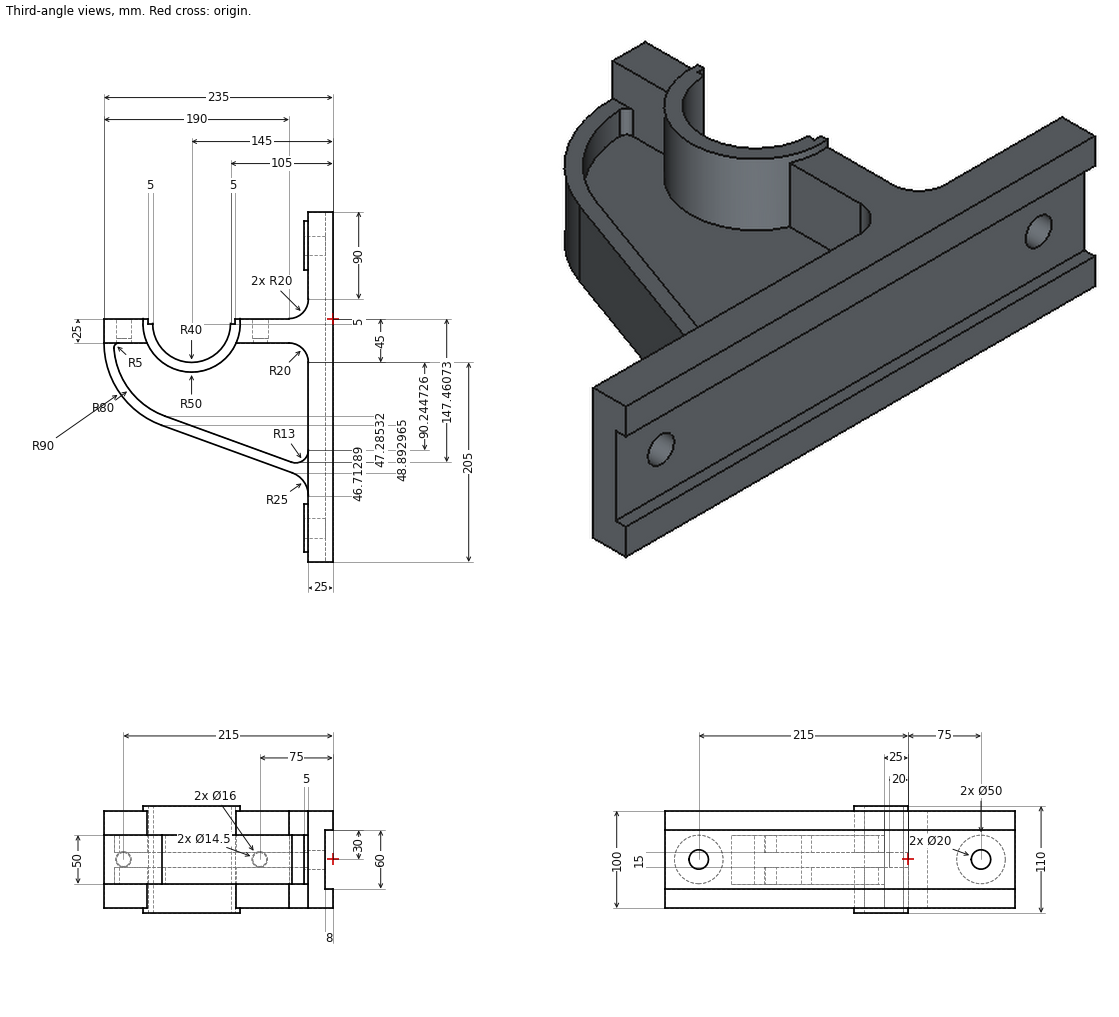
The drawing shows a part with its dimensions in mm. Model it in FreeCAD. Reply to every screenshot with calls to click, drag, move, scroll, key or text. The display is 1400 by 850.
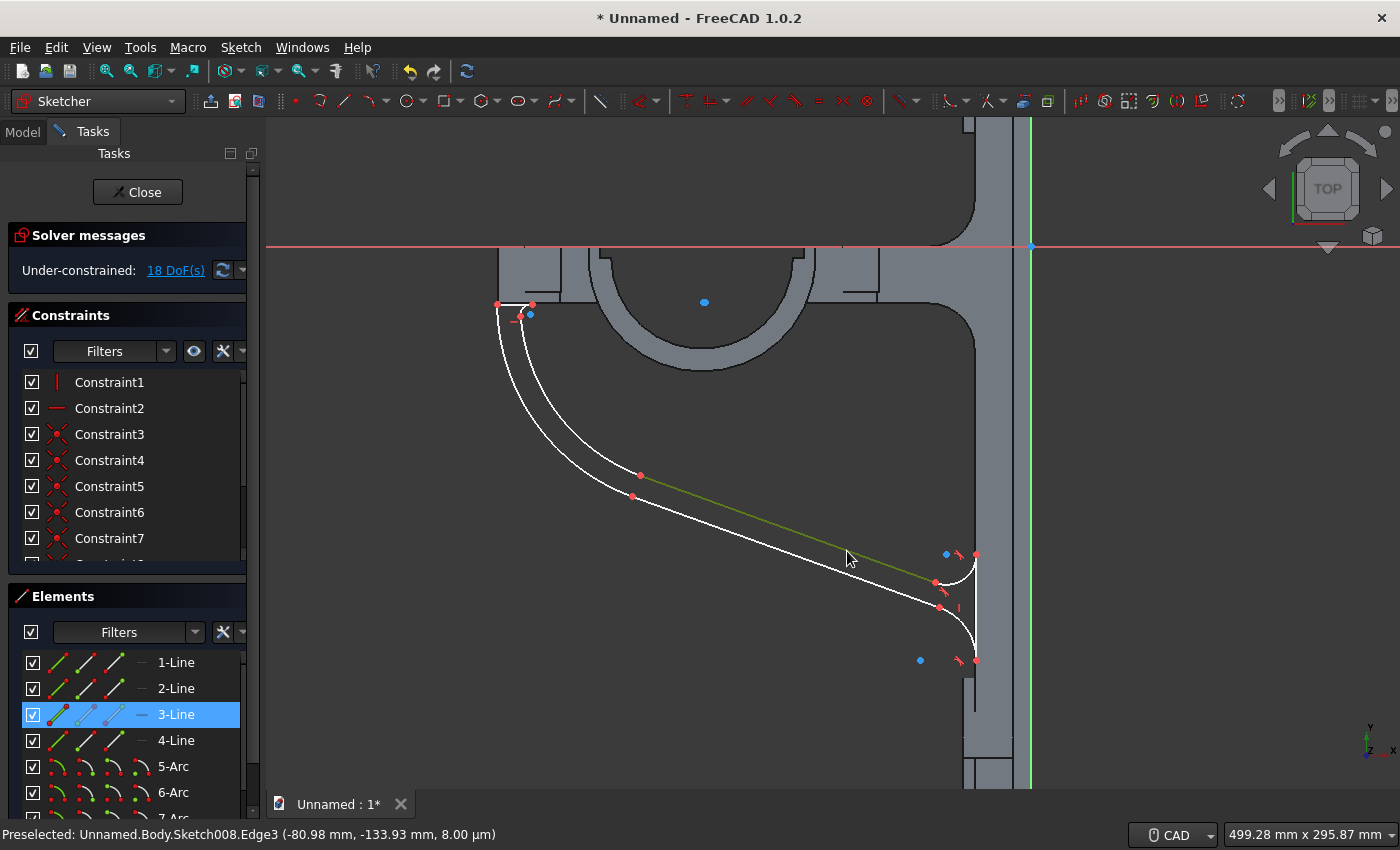
click(952, 584)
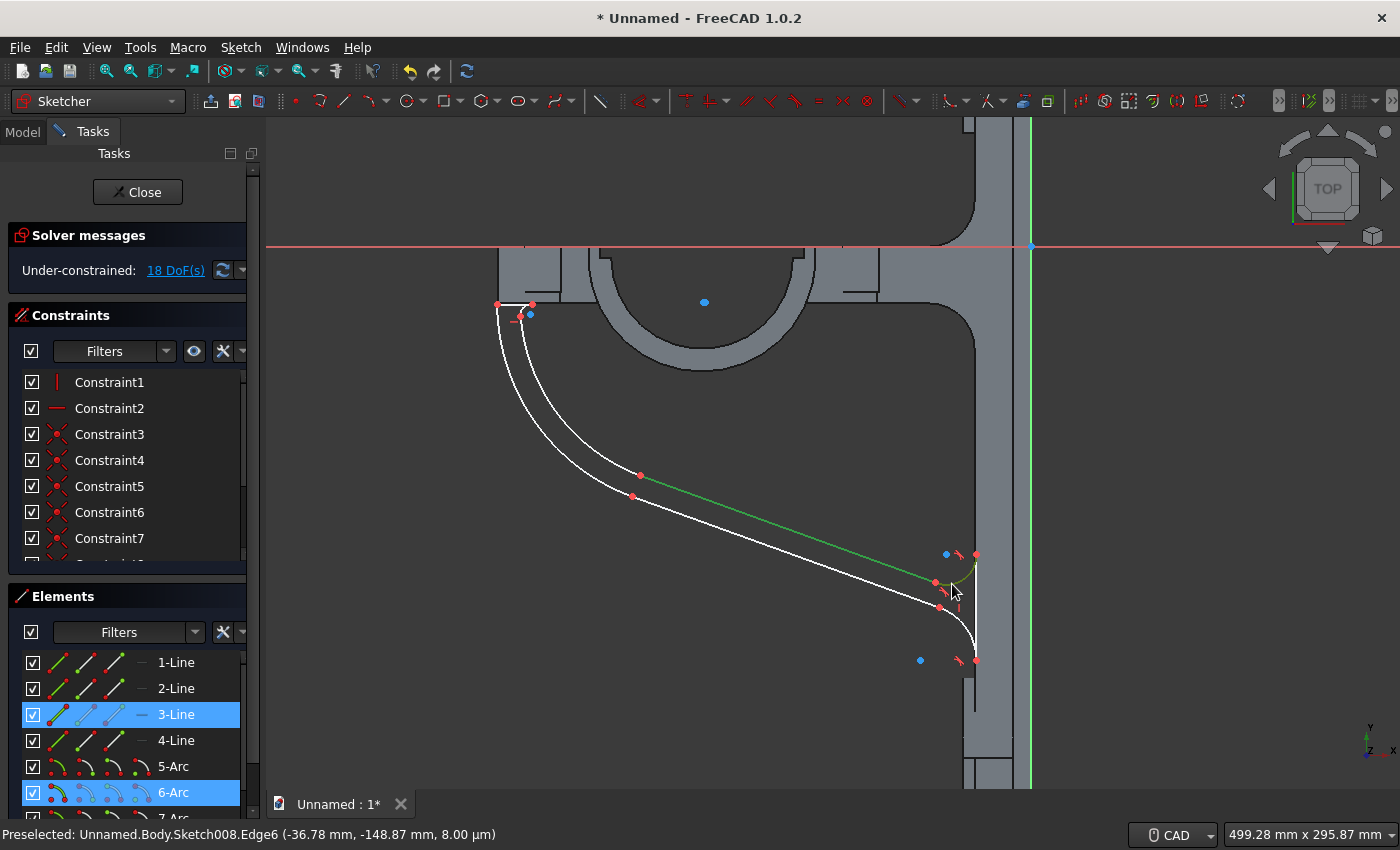
click(796, 102)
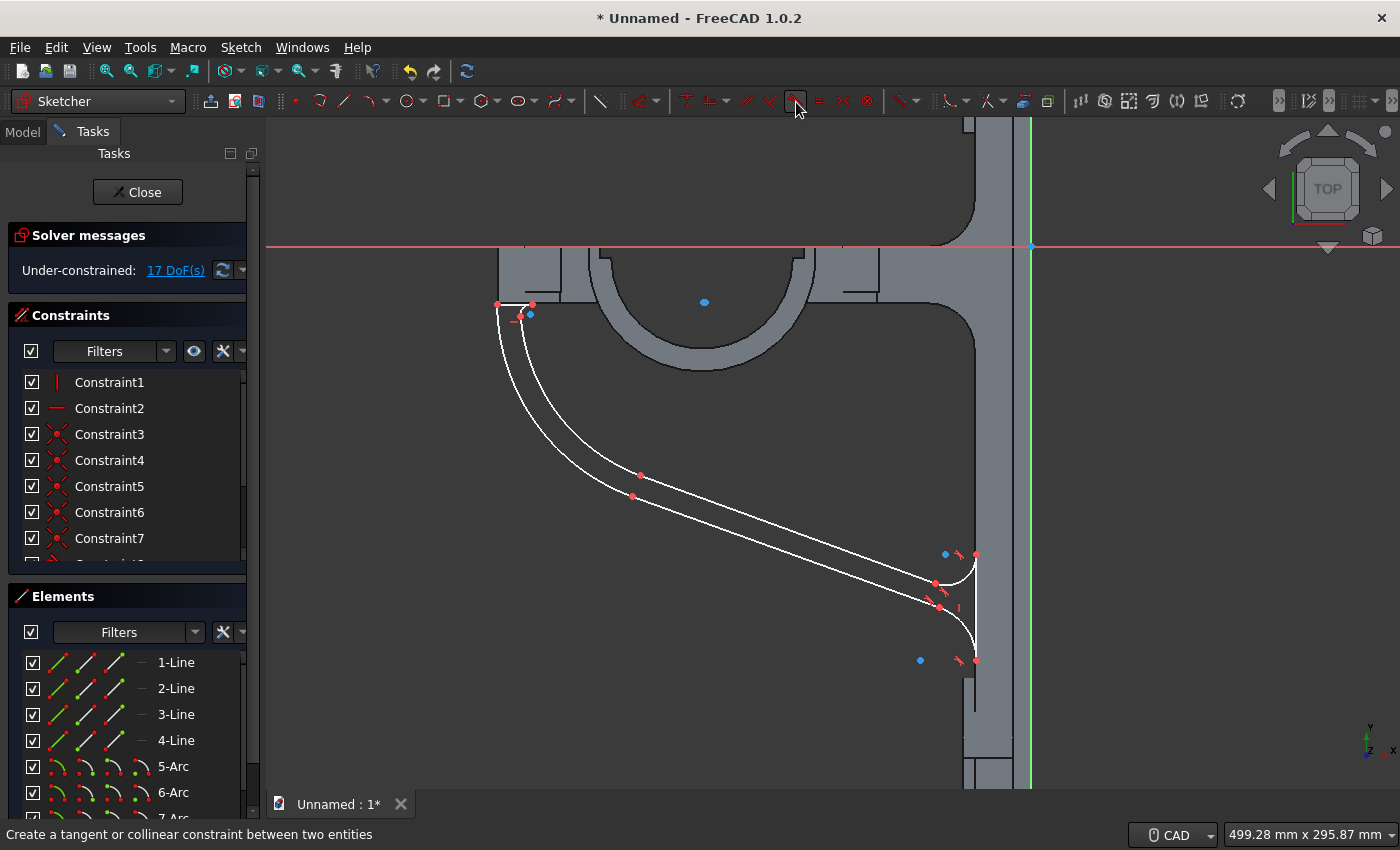
scroll(508, 305, up, 2)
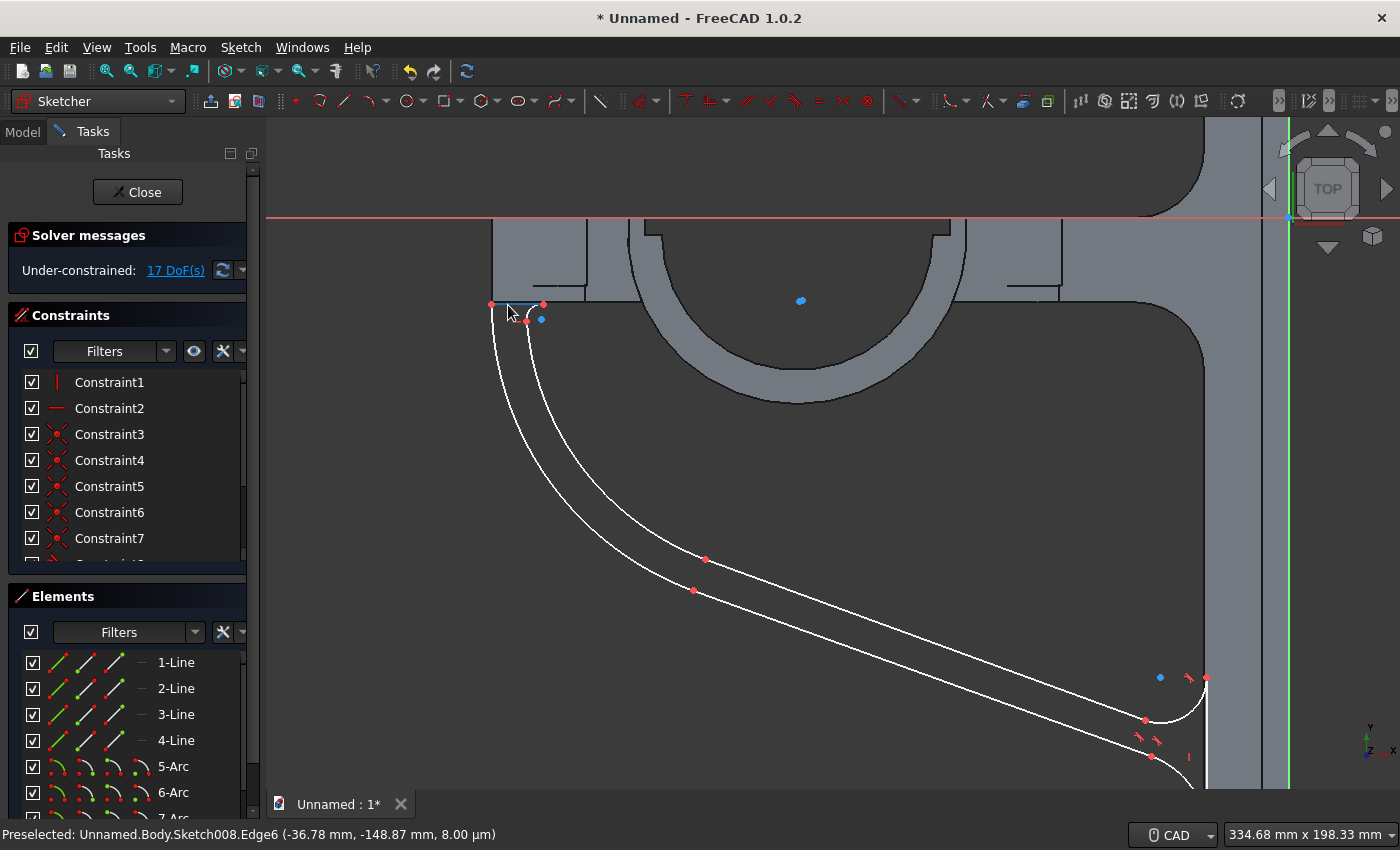
click(507, 304)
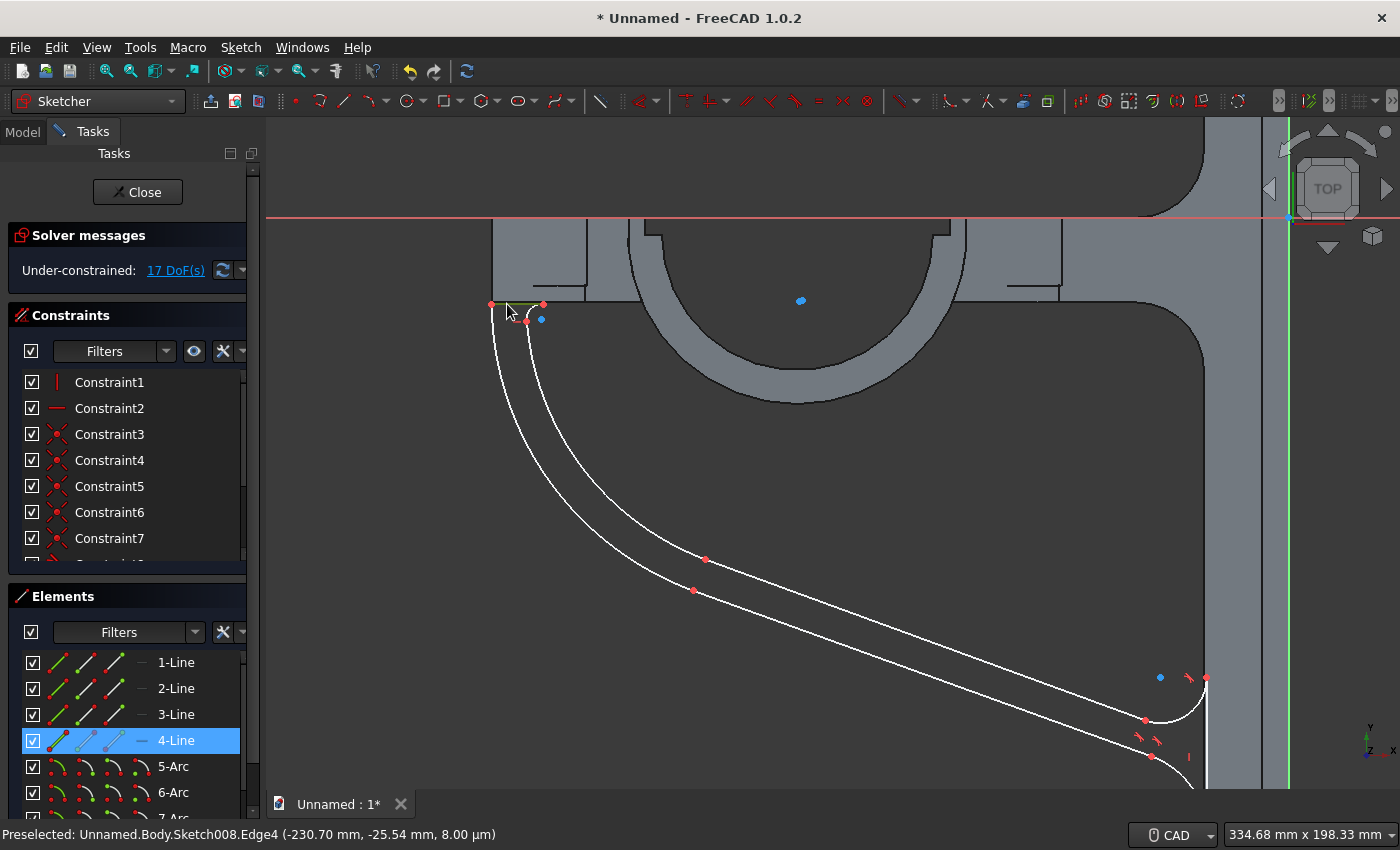
scroll(528, 314, up, 3)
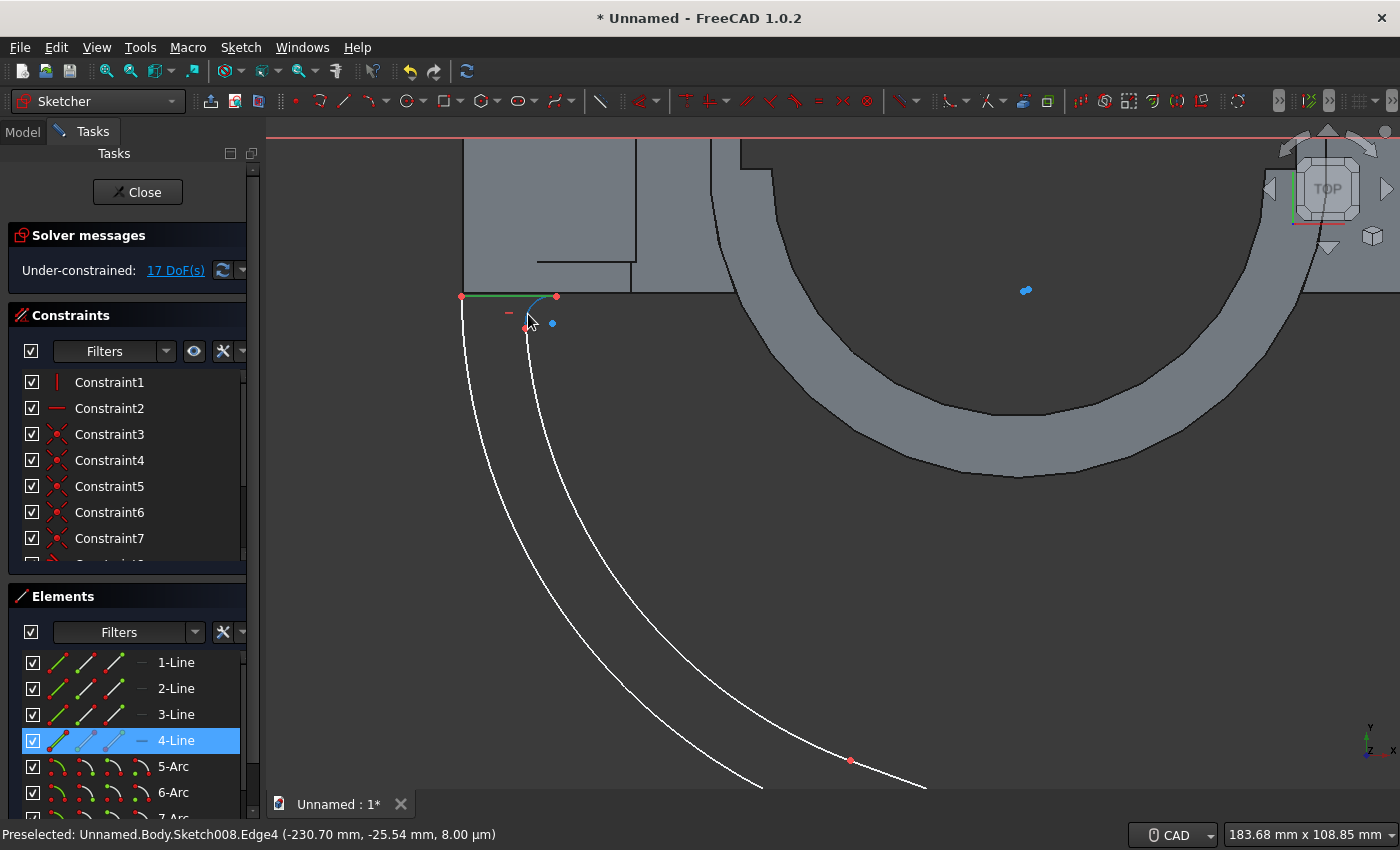
click(527, 313)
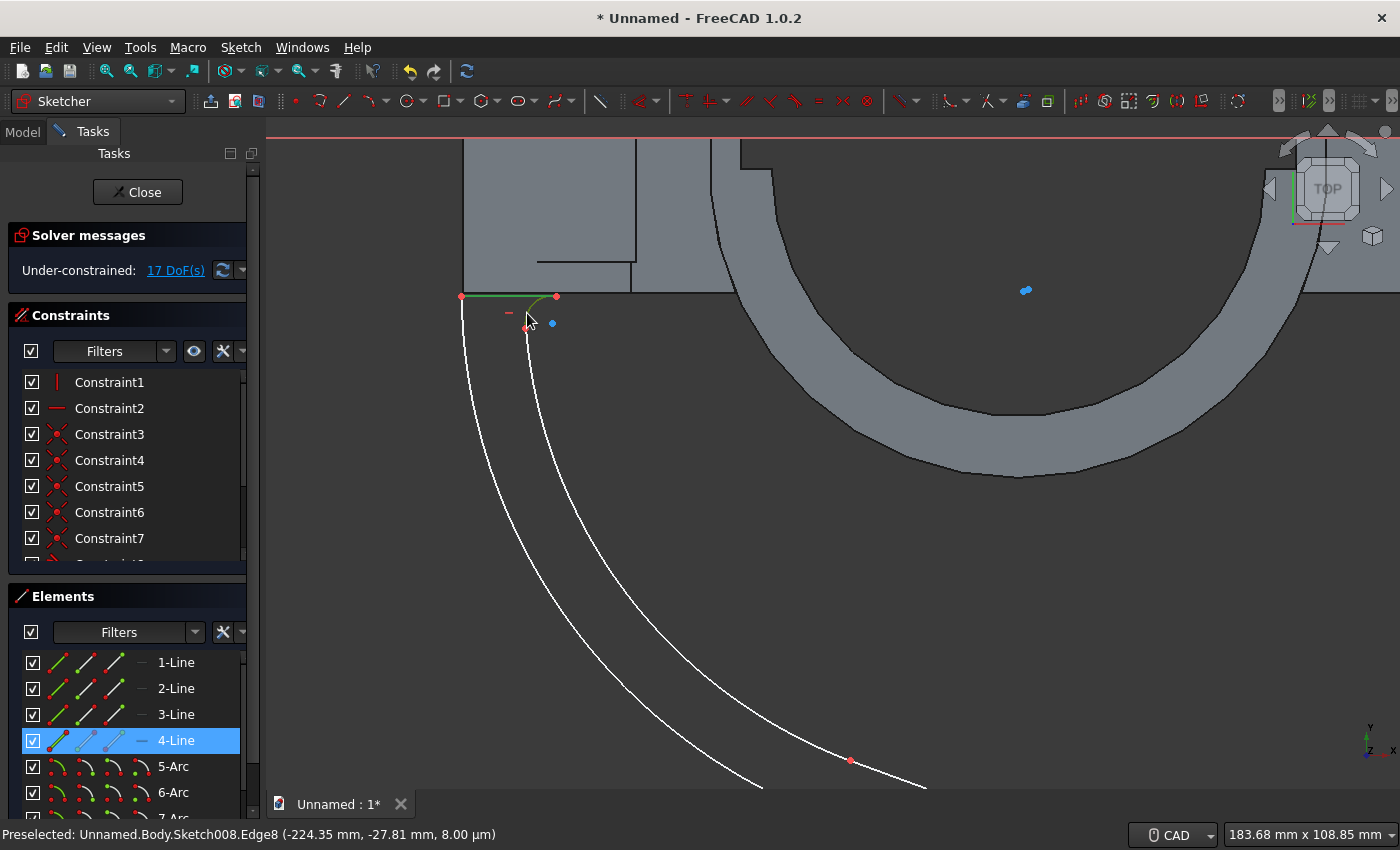
click(796, 102)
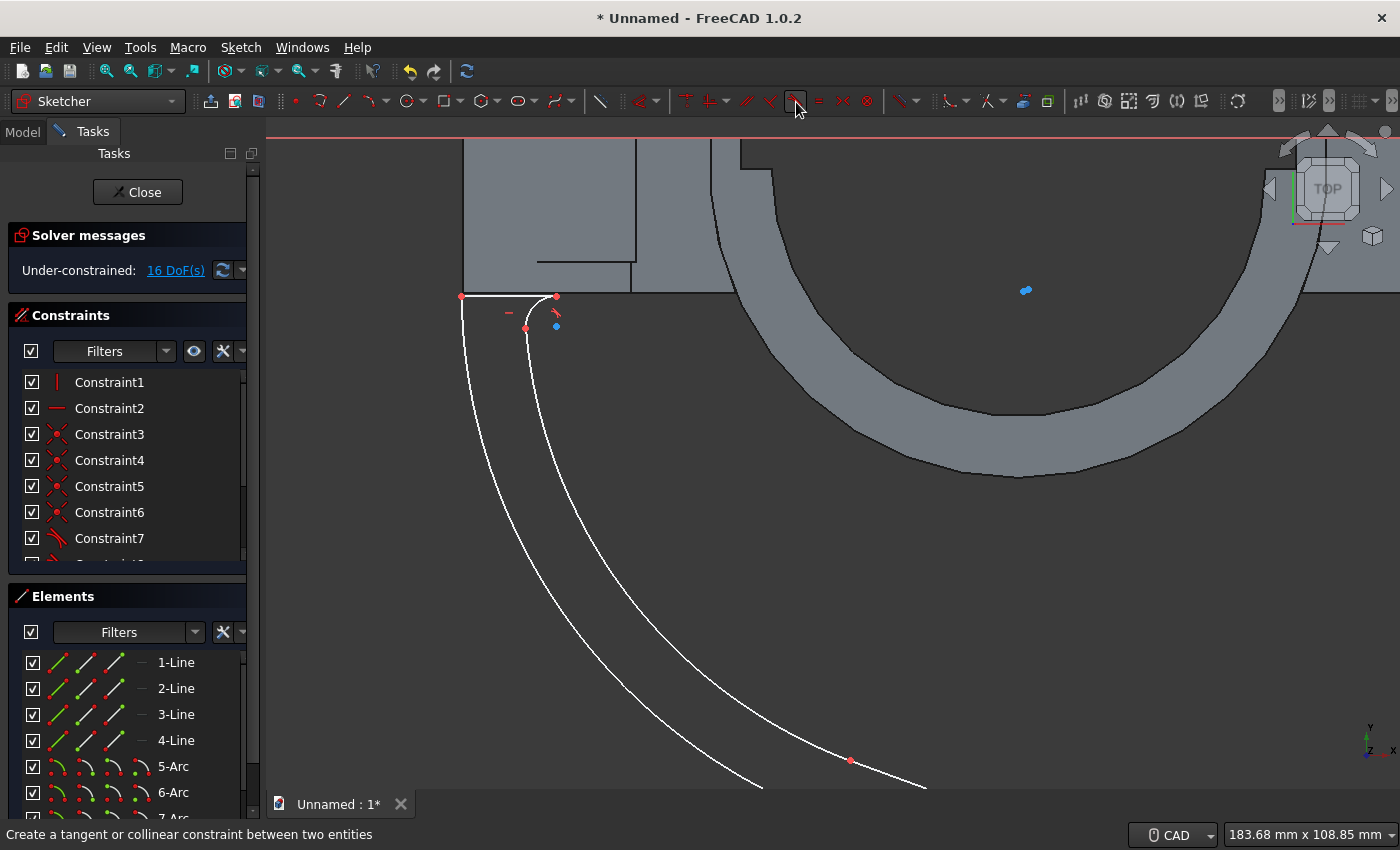
click(568, 494)